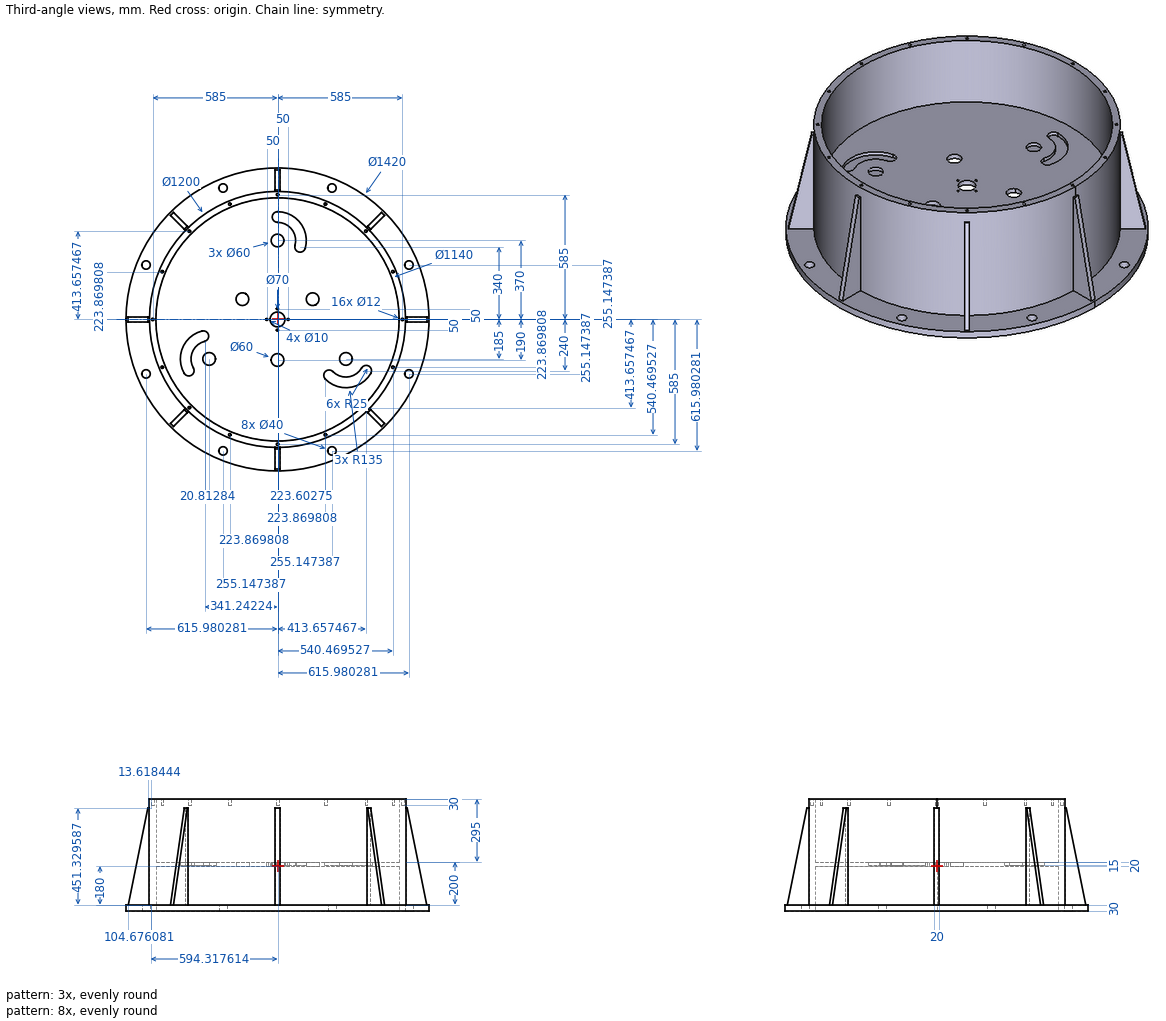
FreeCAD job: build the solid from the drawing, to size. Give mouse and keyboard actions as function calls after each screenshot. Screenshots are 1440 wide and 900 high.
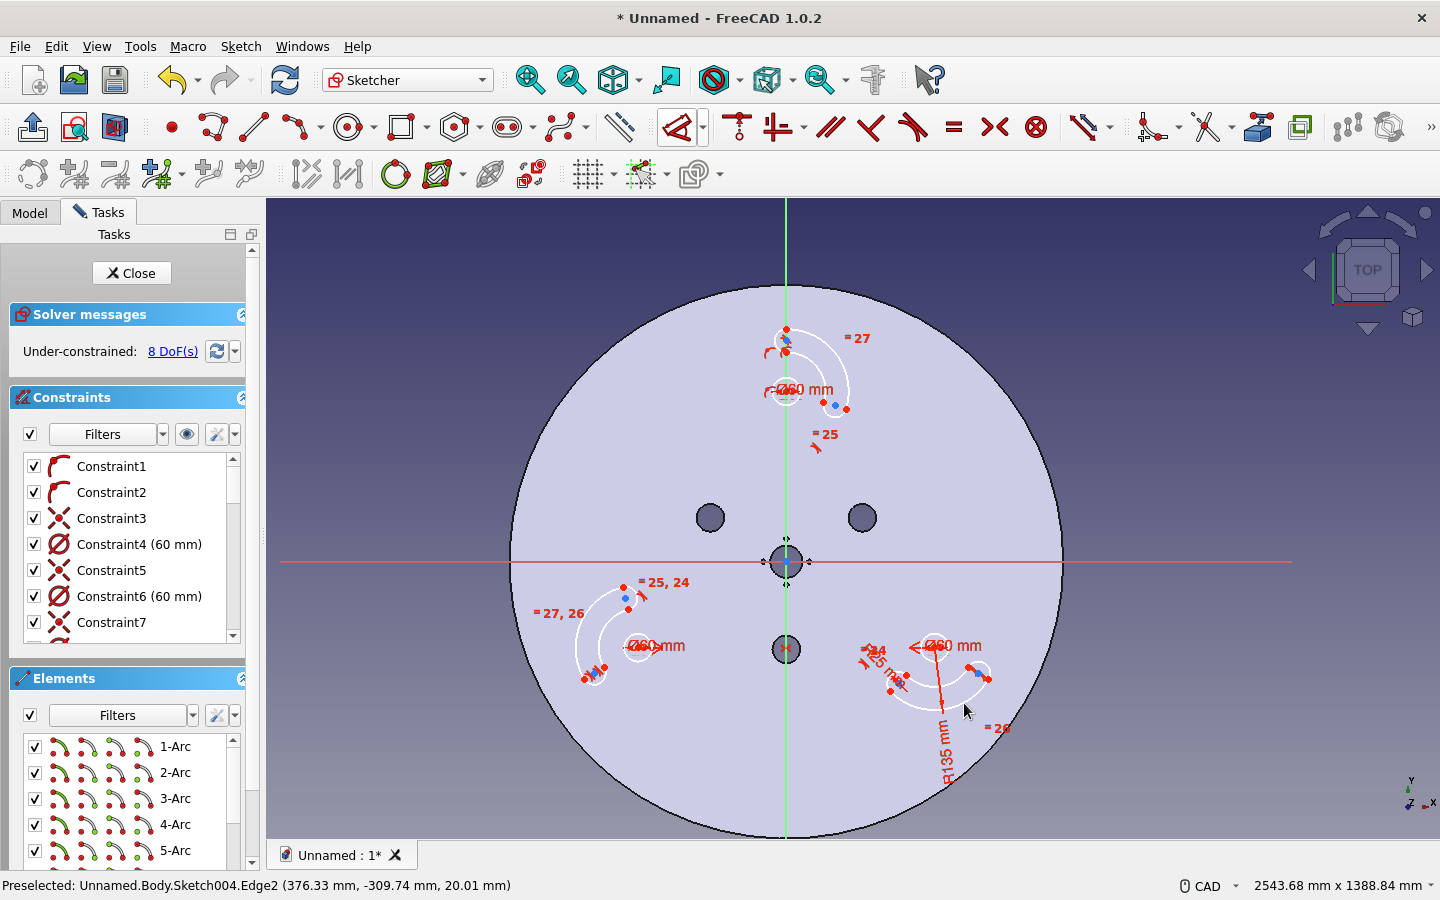
click(786, 392)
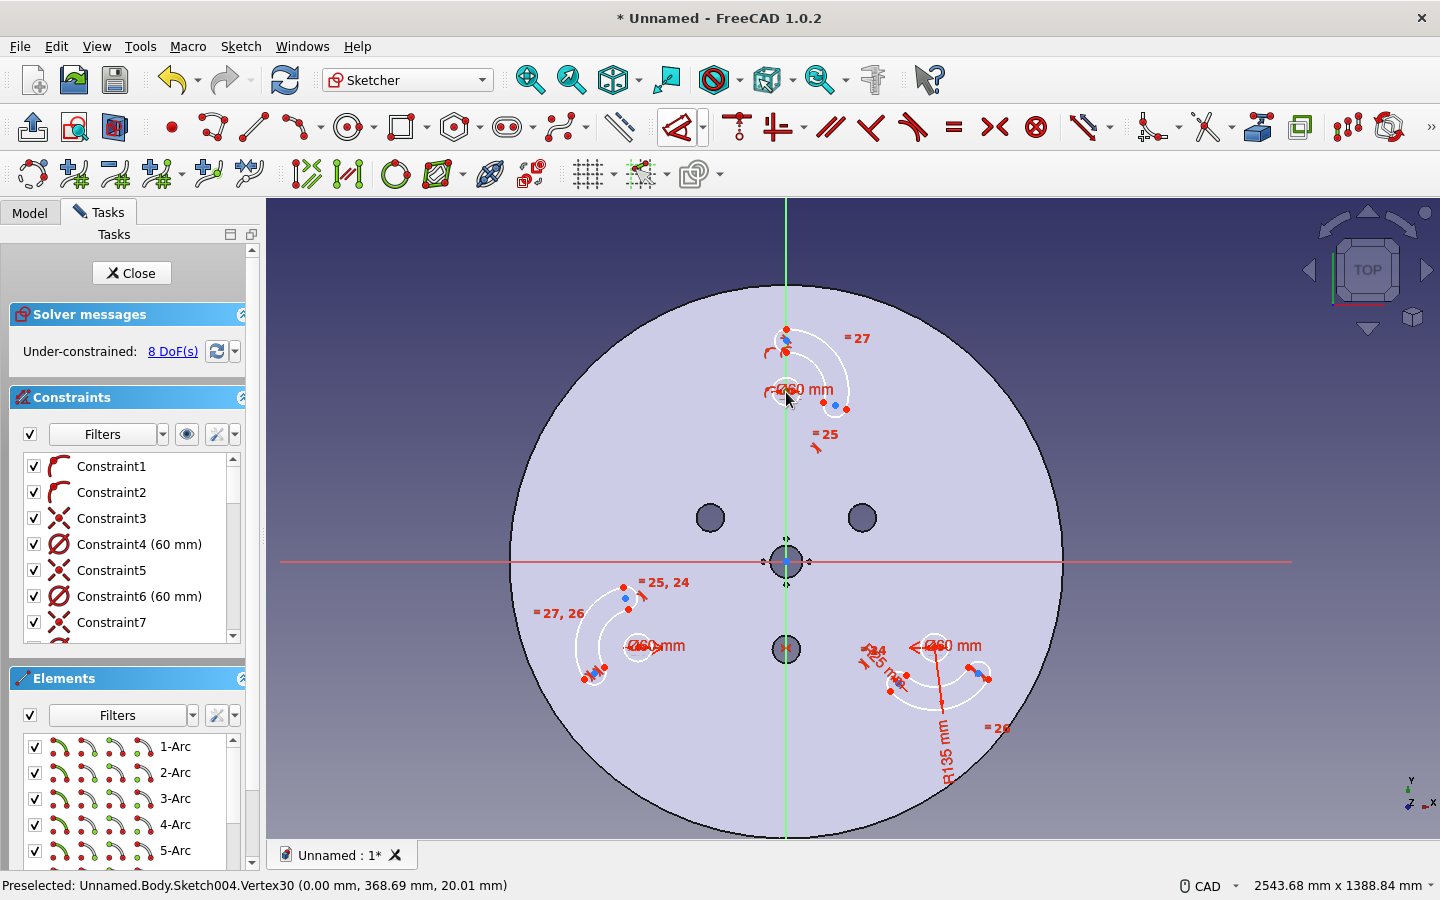
click(702, 128)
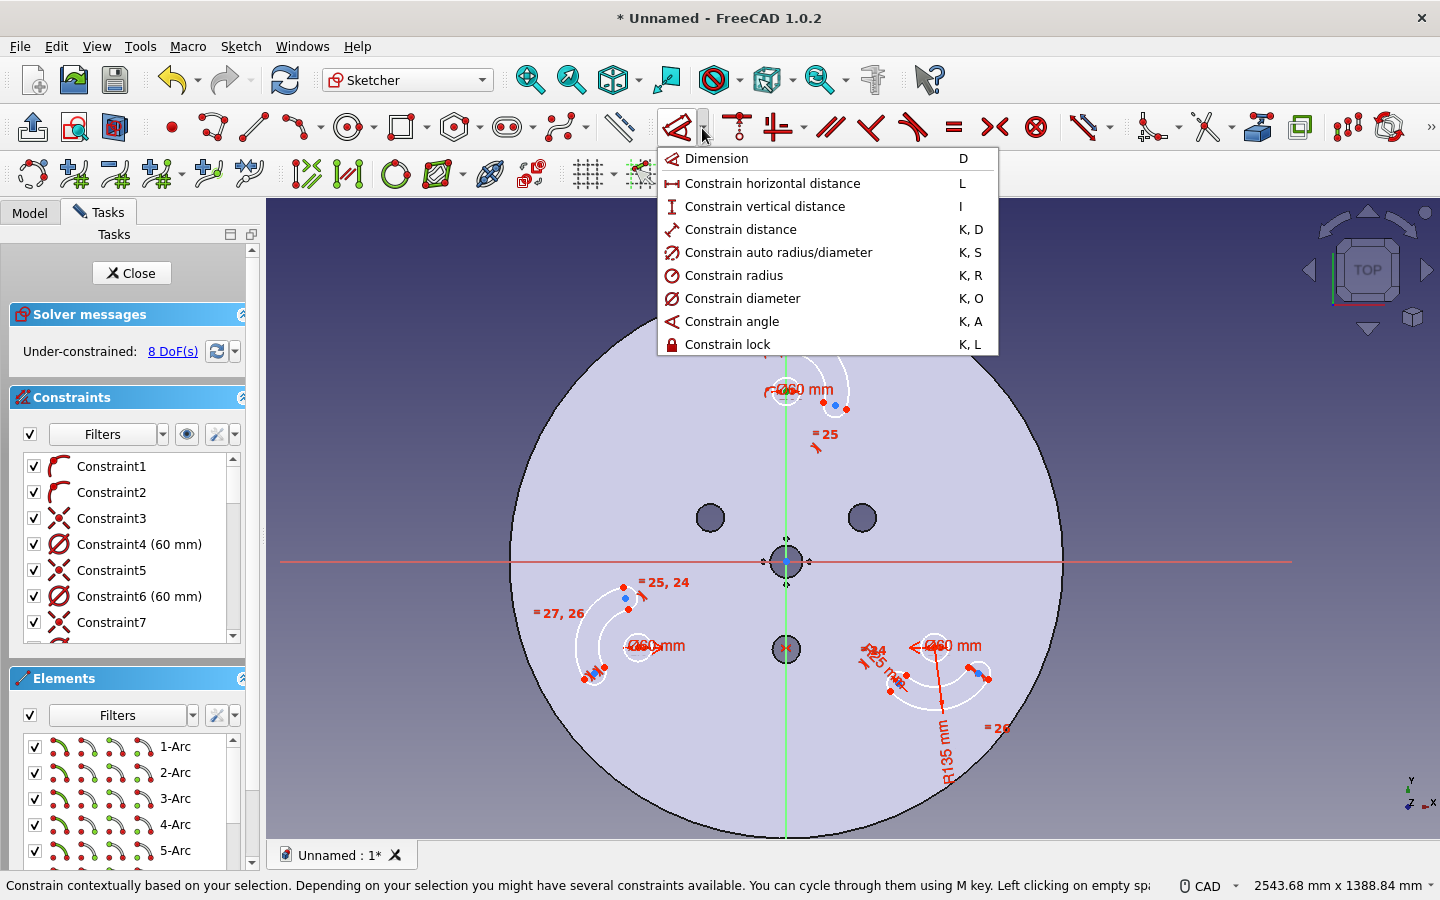
click(828, 206)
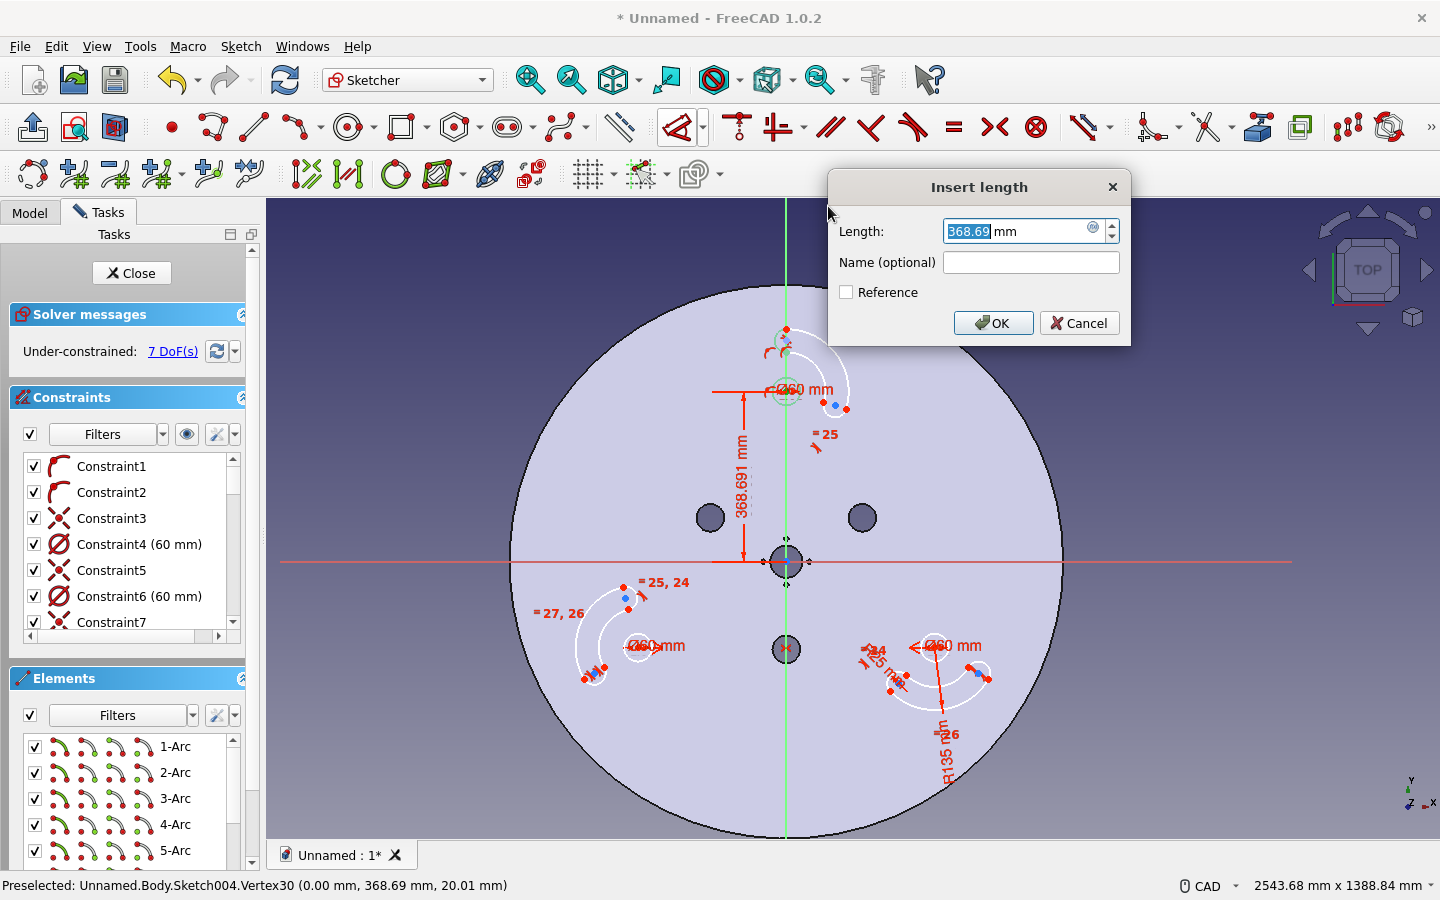
text(370)
key(Return)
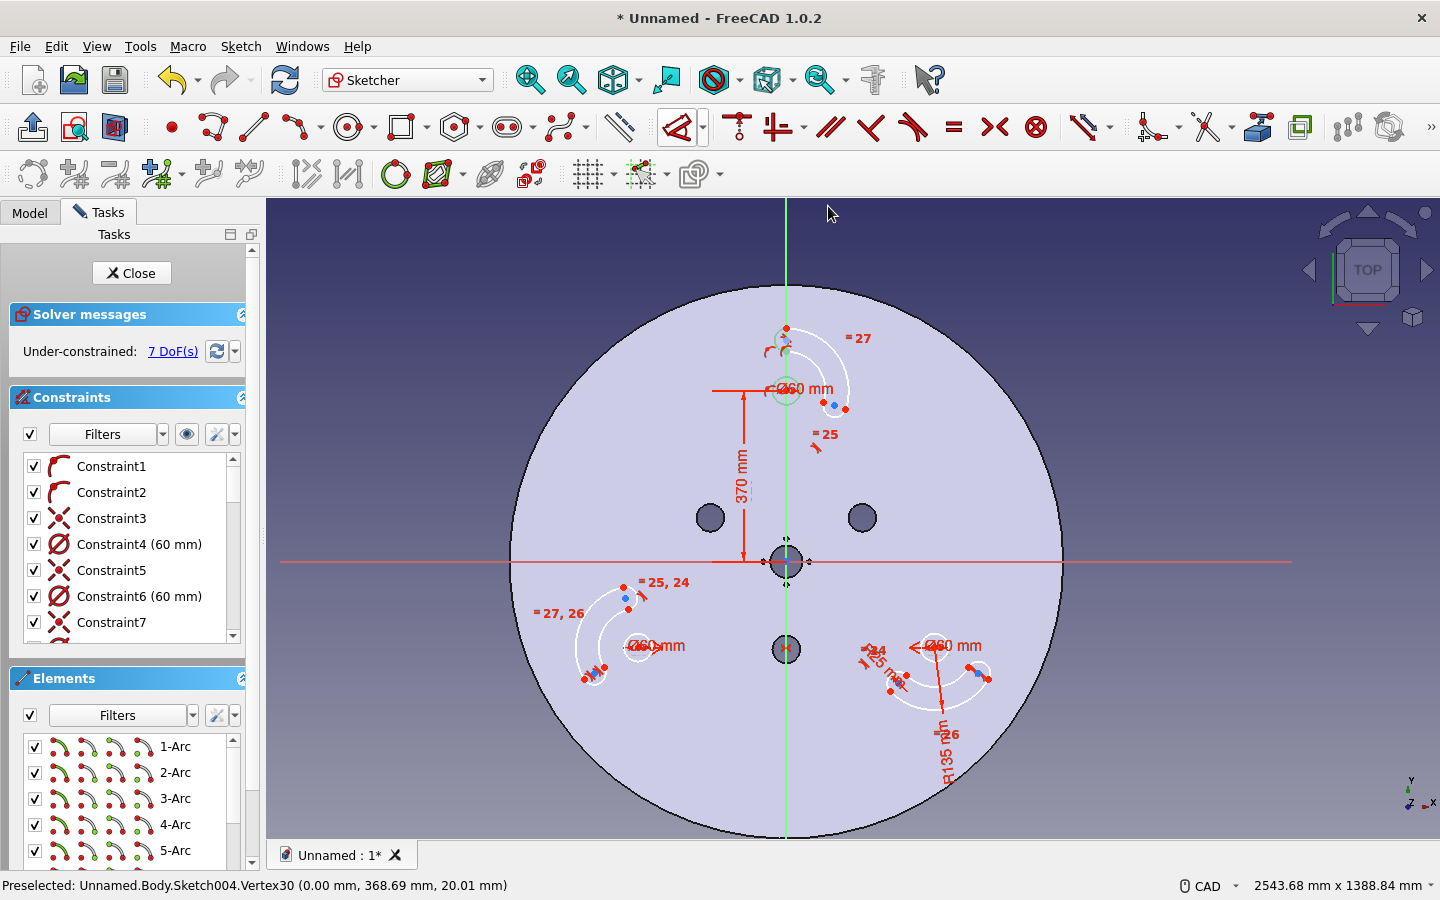
click(935, 648)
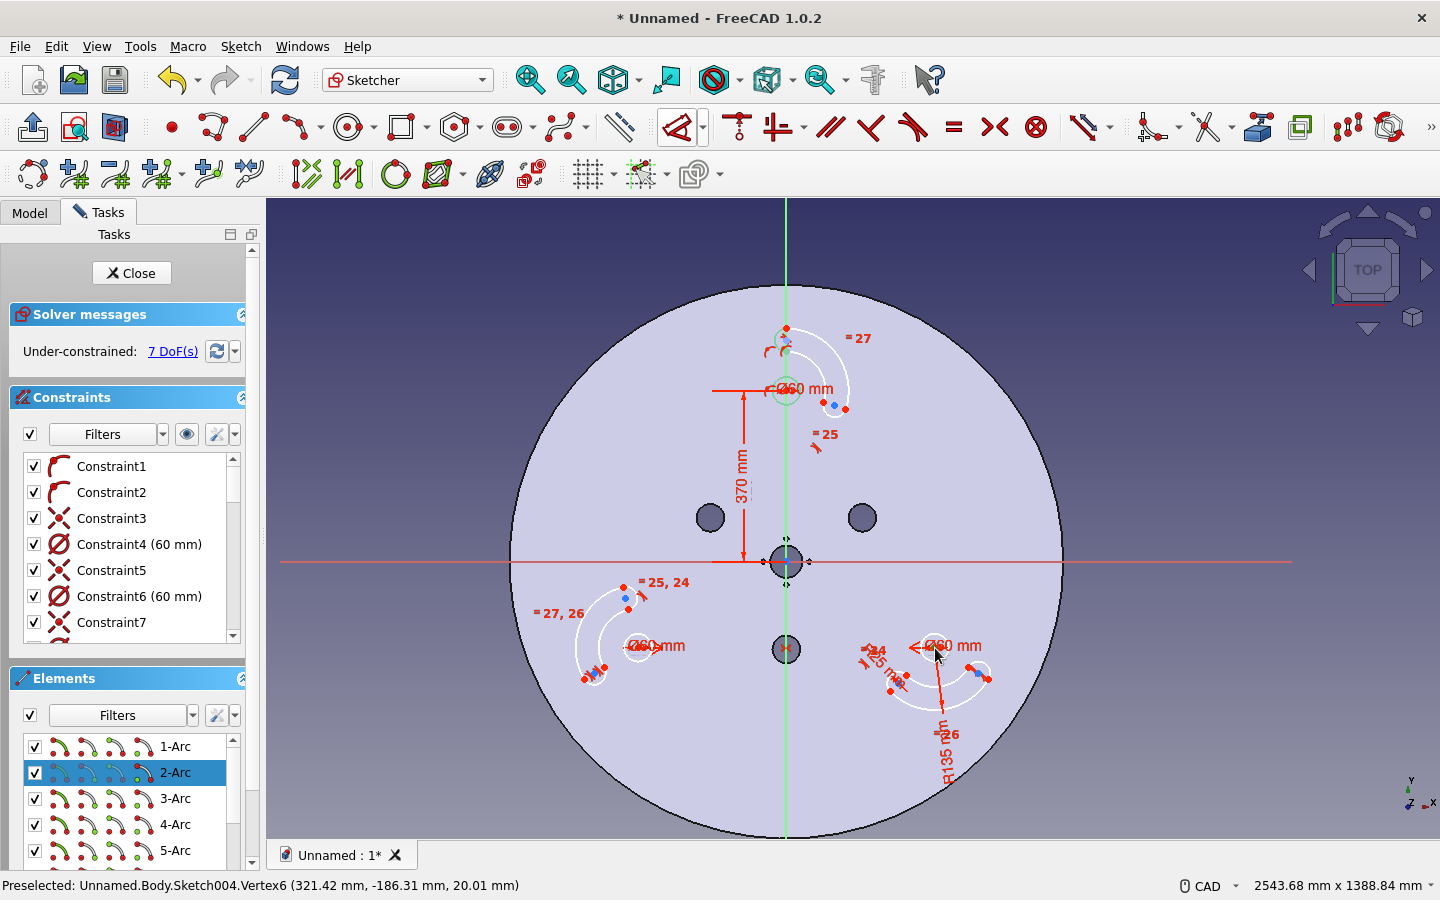
click(702, 128)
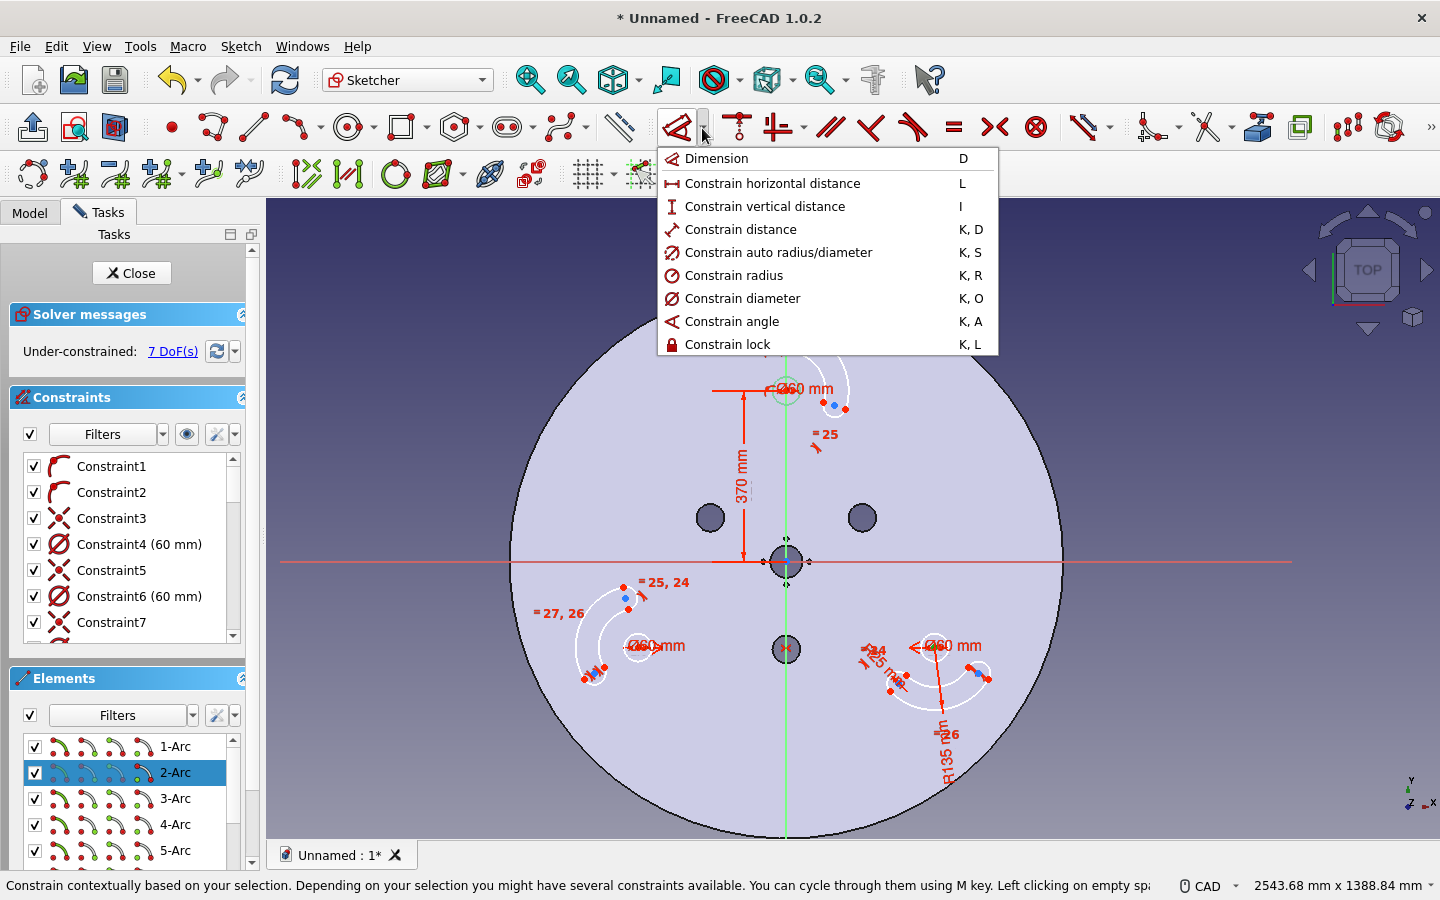
click(828, 206)